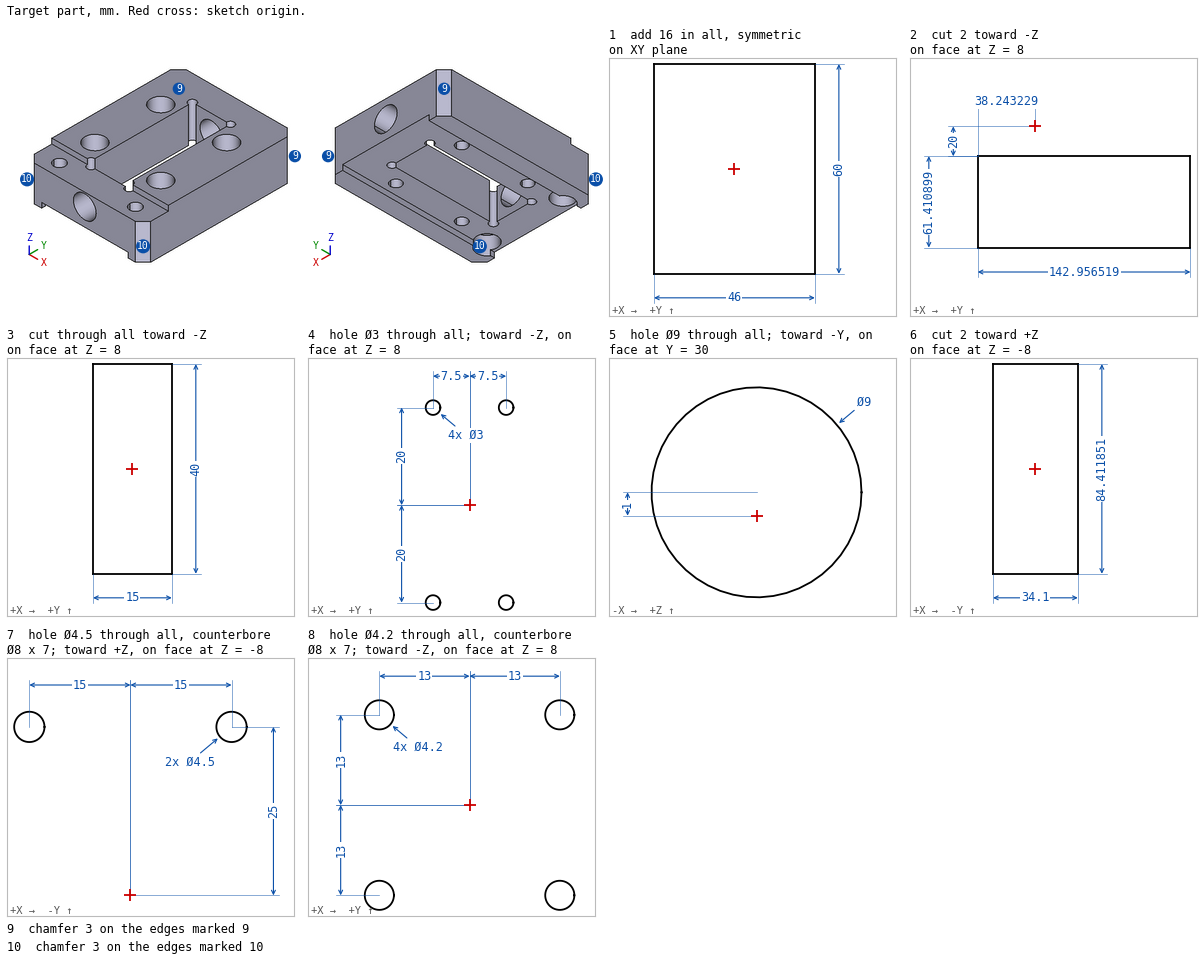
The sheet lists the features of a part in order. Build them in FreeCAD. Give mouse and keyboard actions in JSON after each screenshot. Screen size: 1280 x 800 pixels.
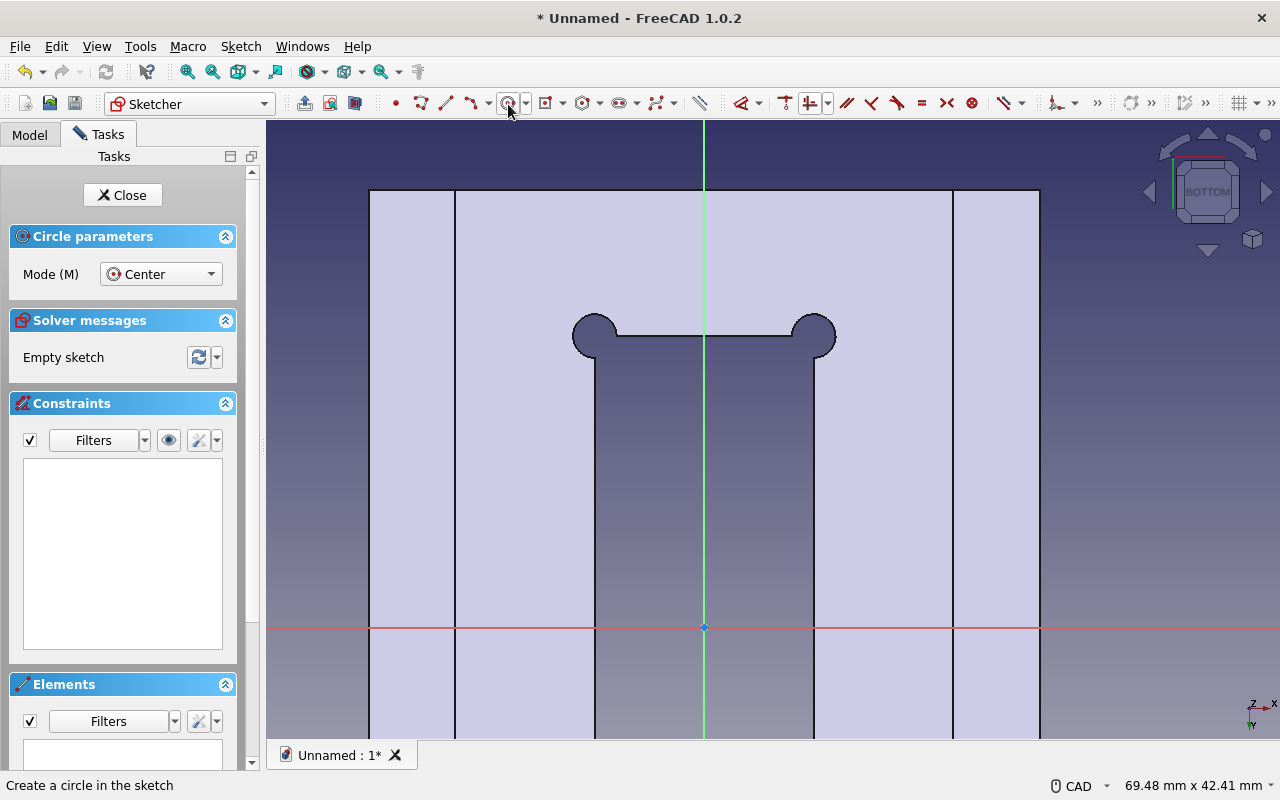
{"action": "left_click", "coordinate": [923, 263]}
{"action": "left_click", "coordinate": [946, 240]}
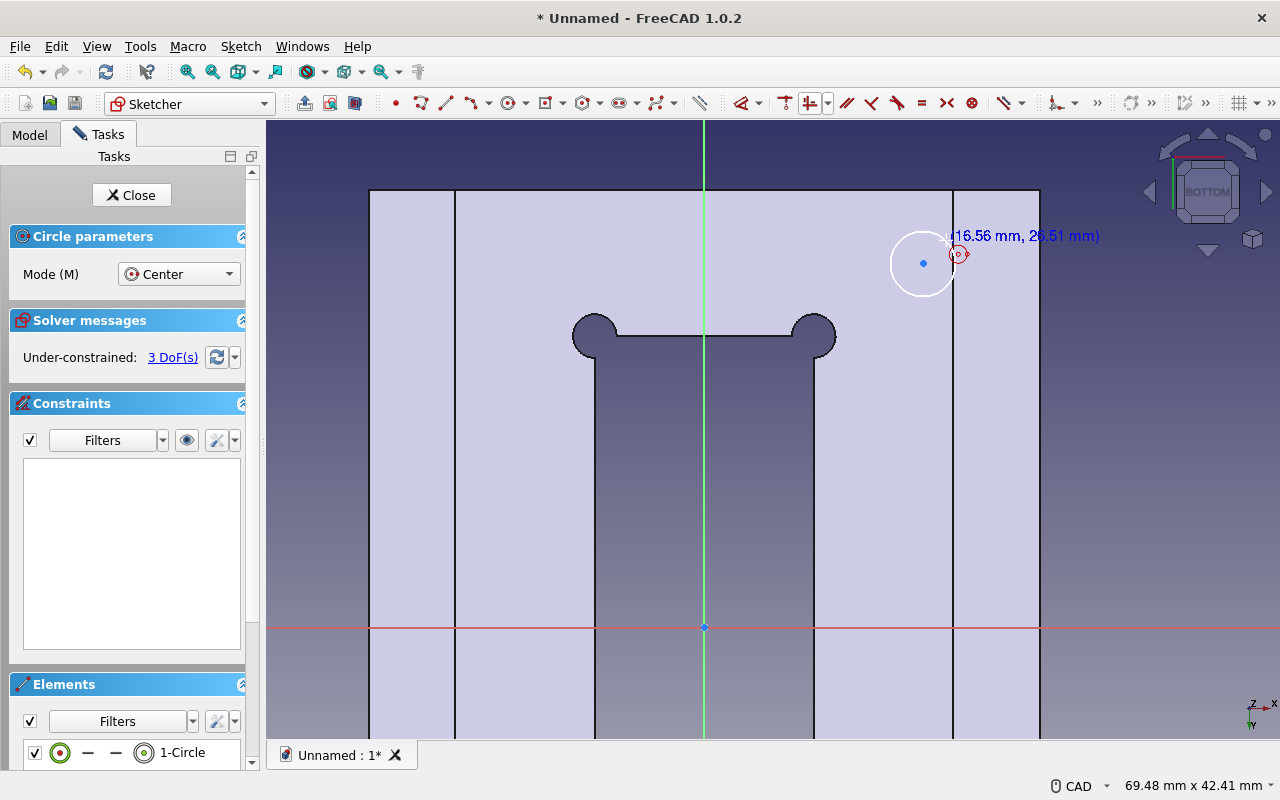
{"action": "left_click", "coordinate": [485, 263]}
{"action": "left_click", "coordinate": [509, 240]}
{"action": "key", "text": "Escape"}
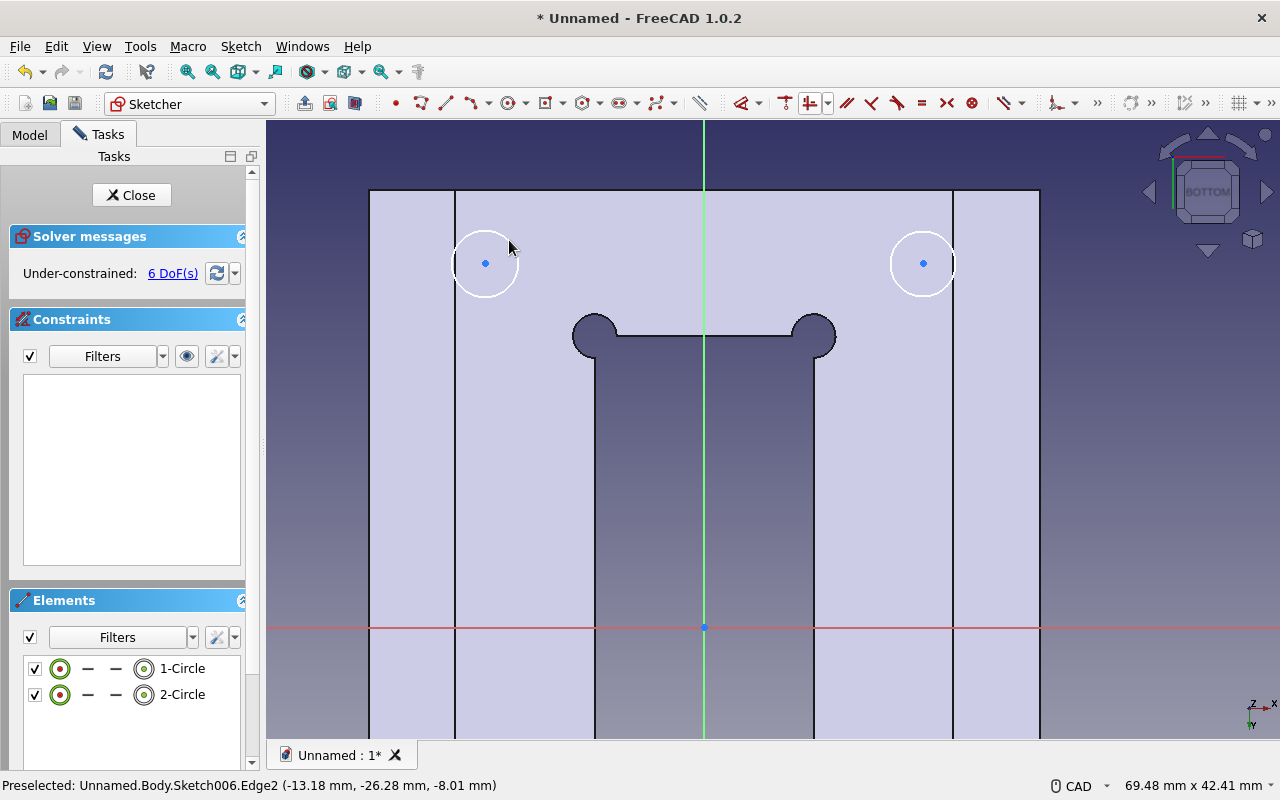
{"action": "left_click", "coordinate": [946, 241]}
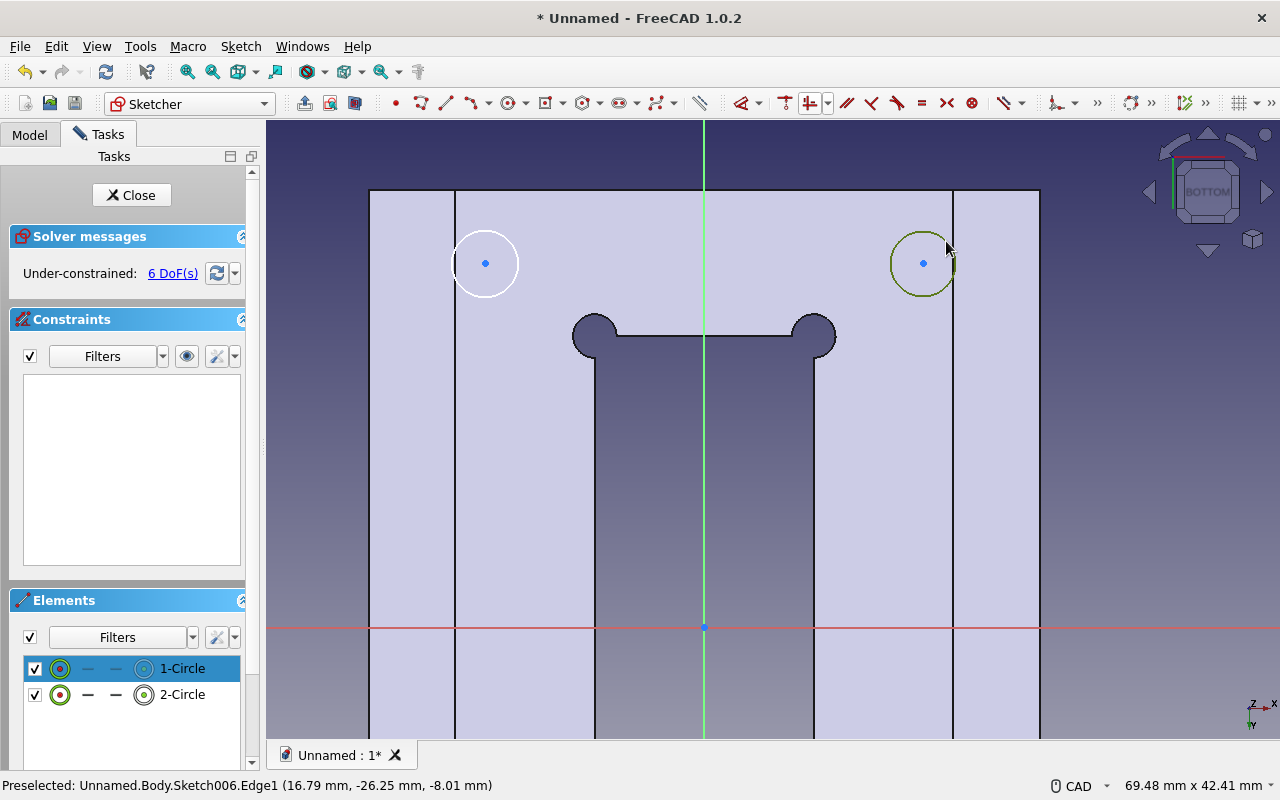
{"action": "left_click", "coordinate": [508, 240]}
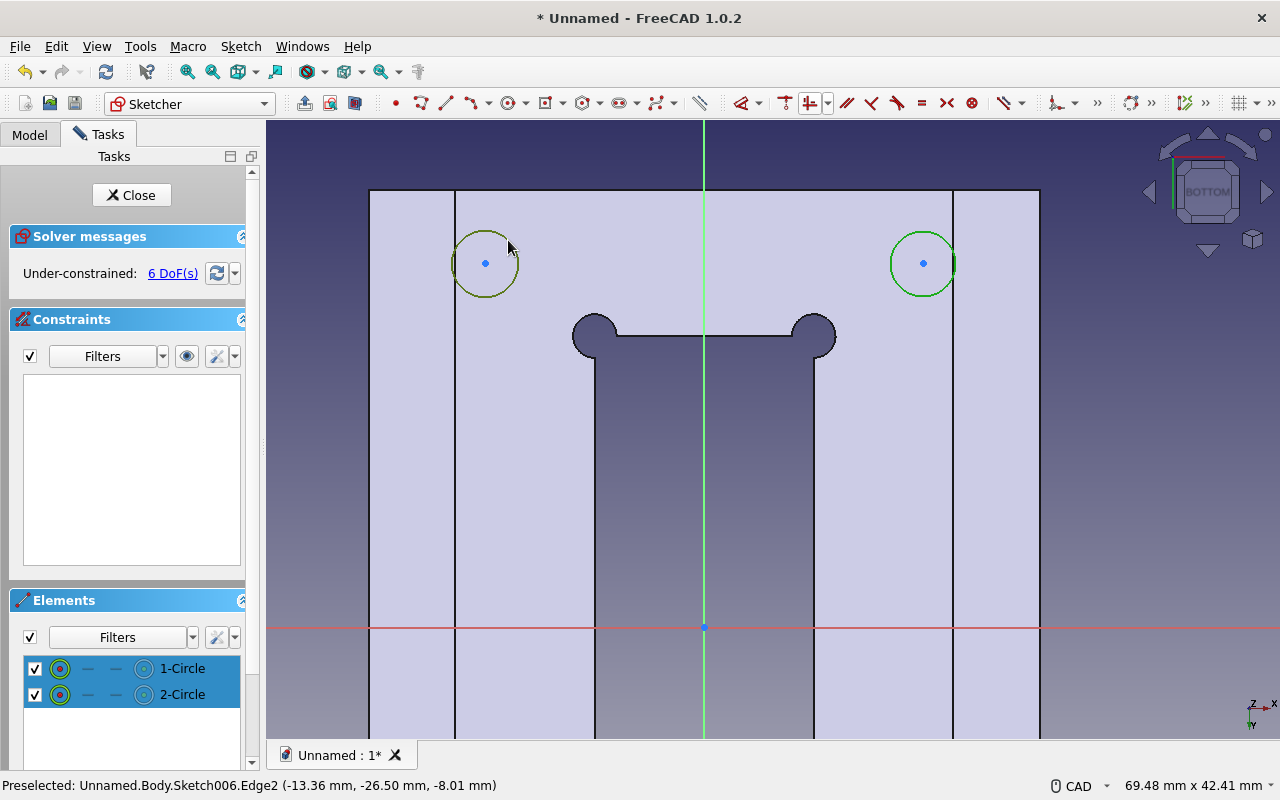
{"action": "left_click", "coordinate": [922, 104]}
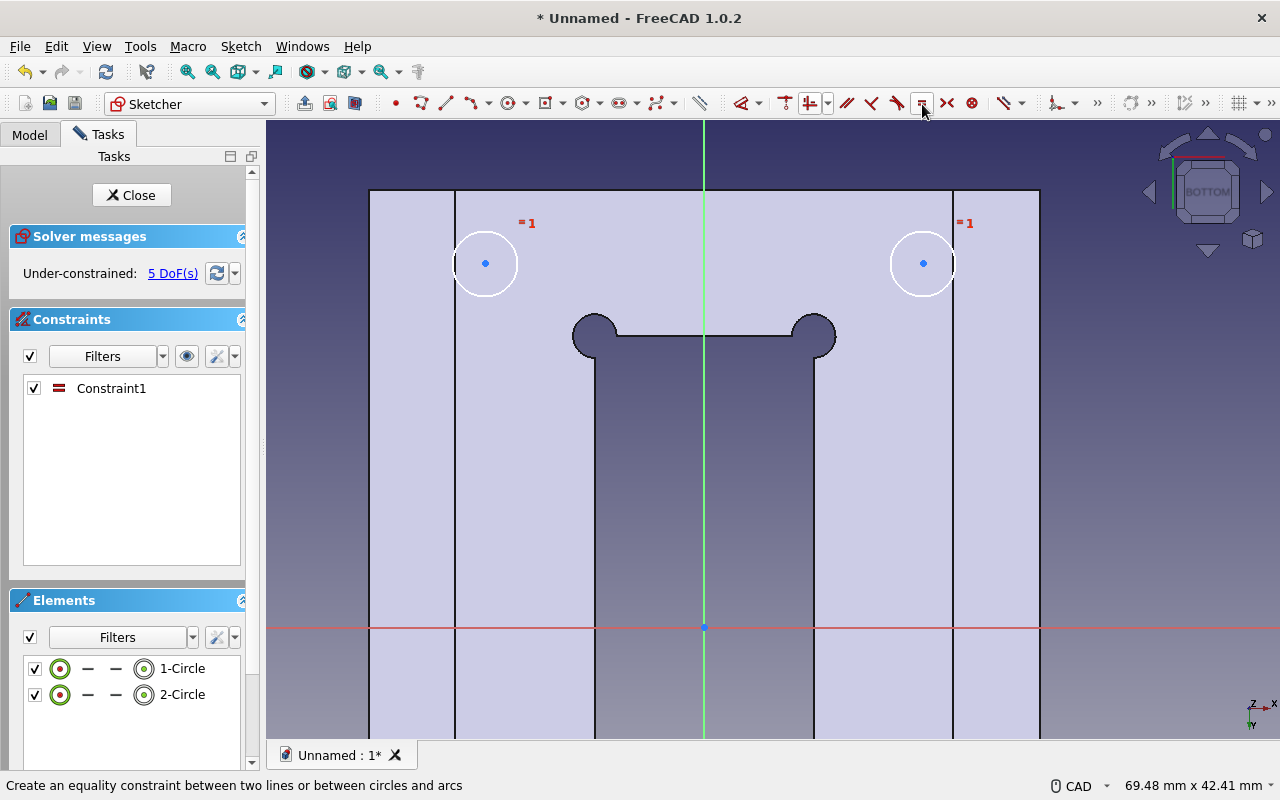
{"action": "left_click", "coordinate": [923, 264]}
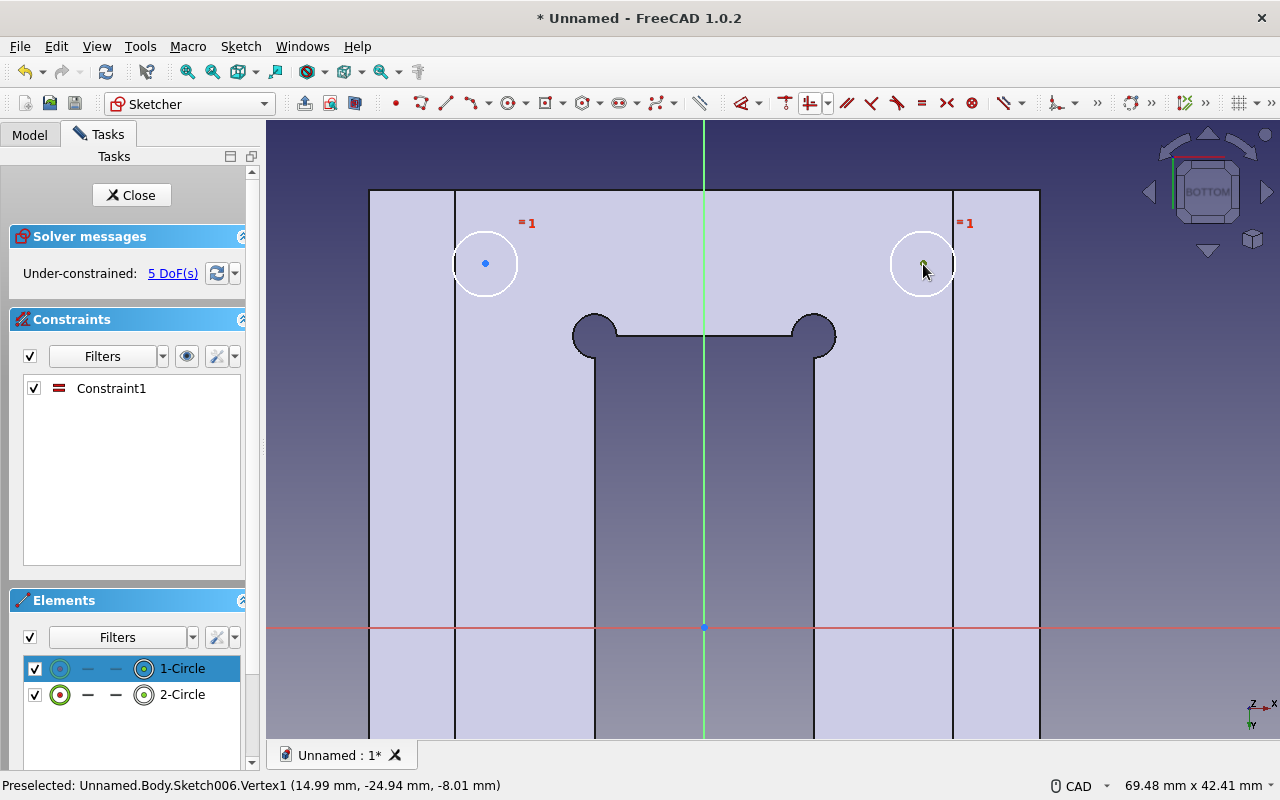
{"action": "left_click", "coordinate": [485, 264]}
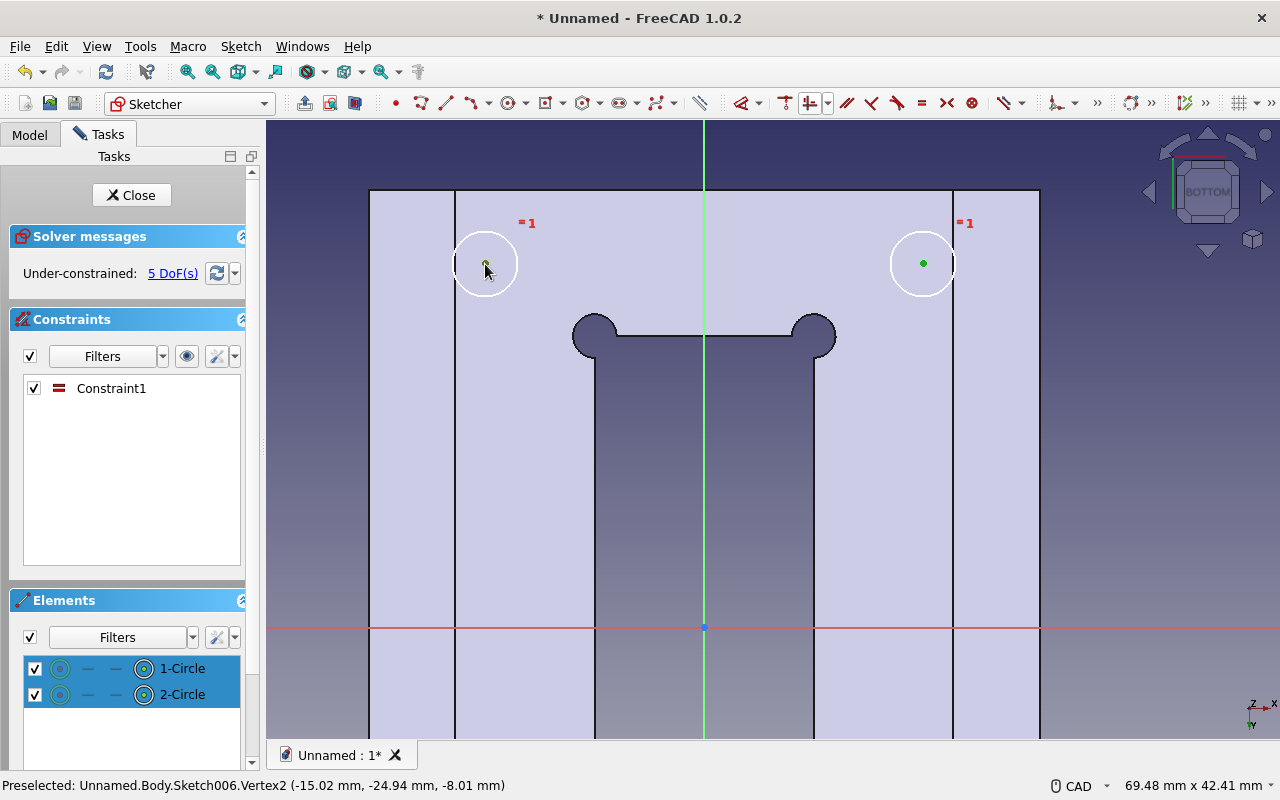
{"action": "left_click", "coordinate": [828, 104]}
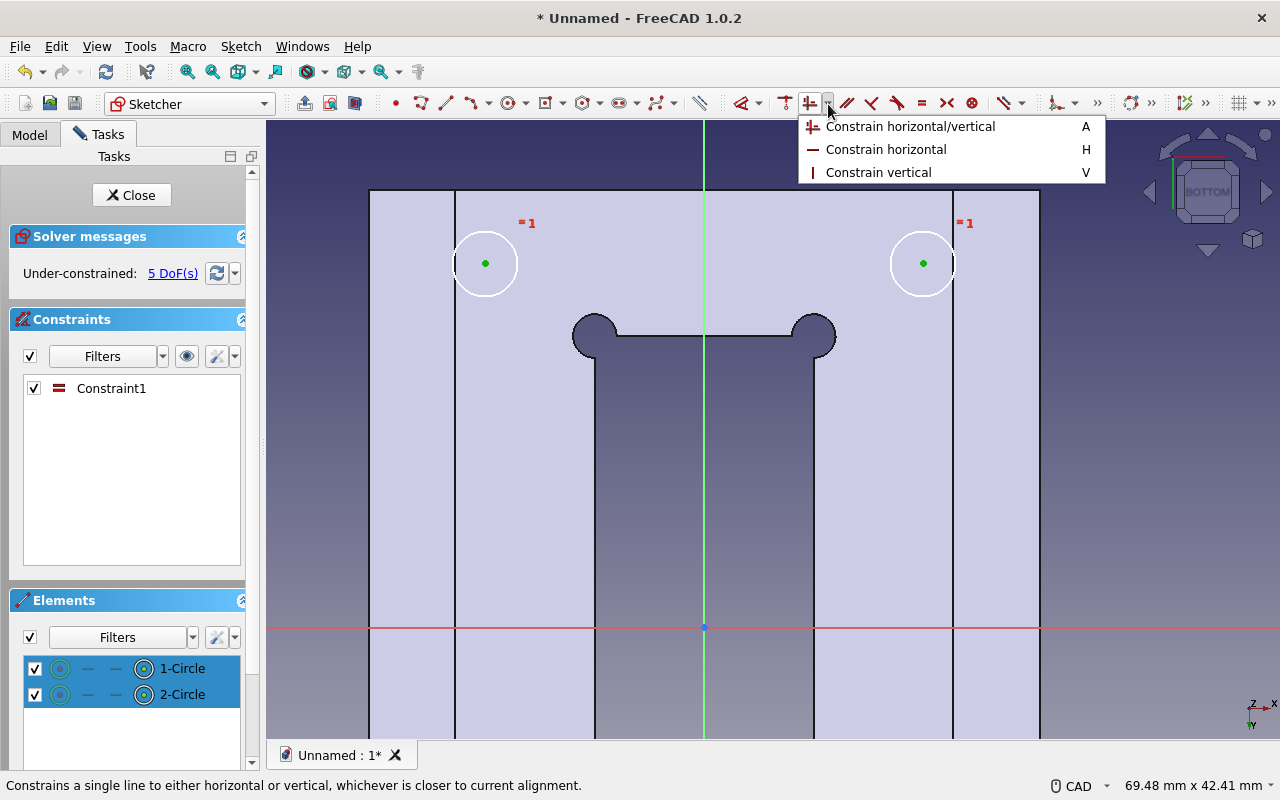
{"action": "left_click", "coordinate": [952, 150]}